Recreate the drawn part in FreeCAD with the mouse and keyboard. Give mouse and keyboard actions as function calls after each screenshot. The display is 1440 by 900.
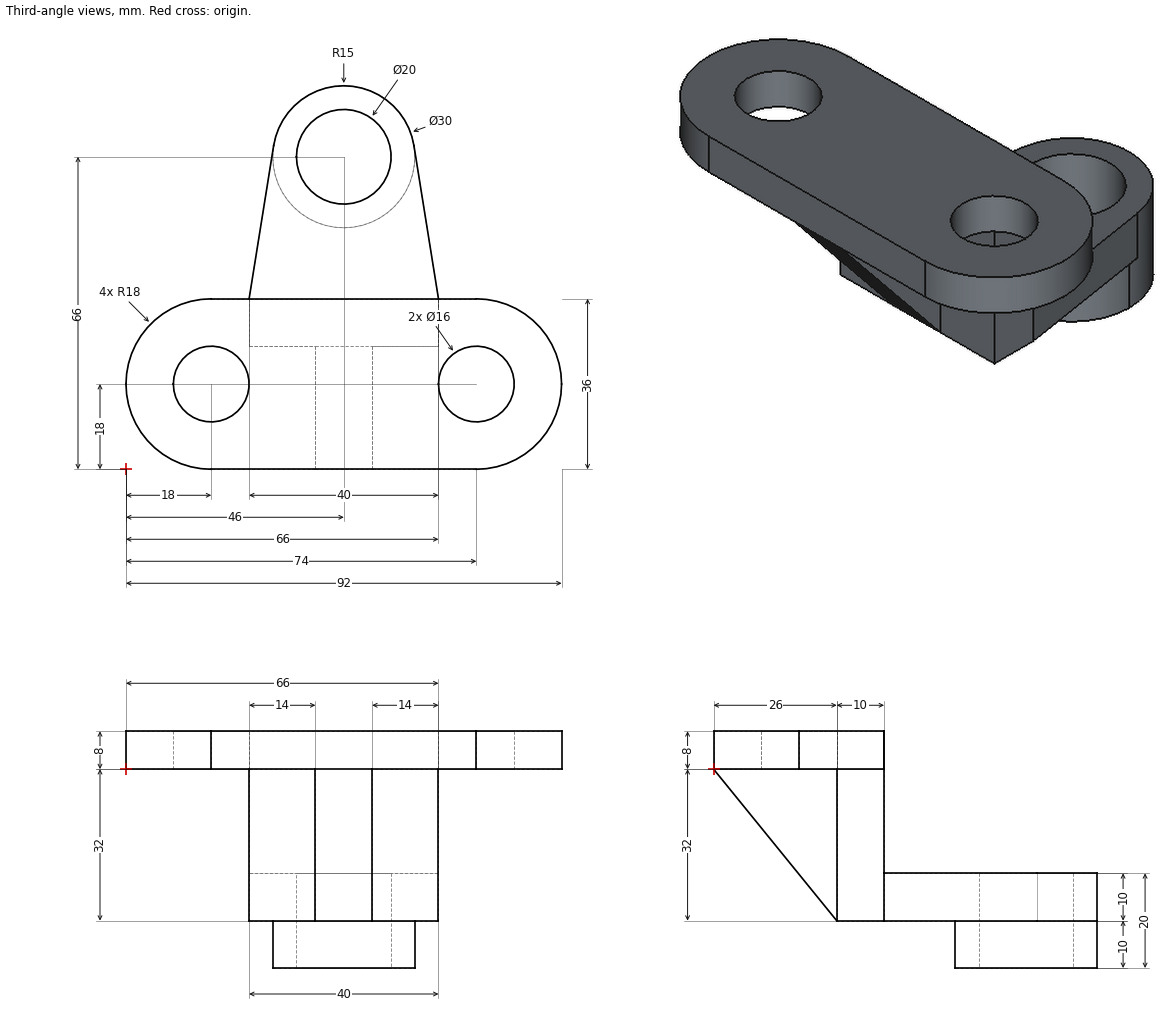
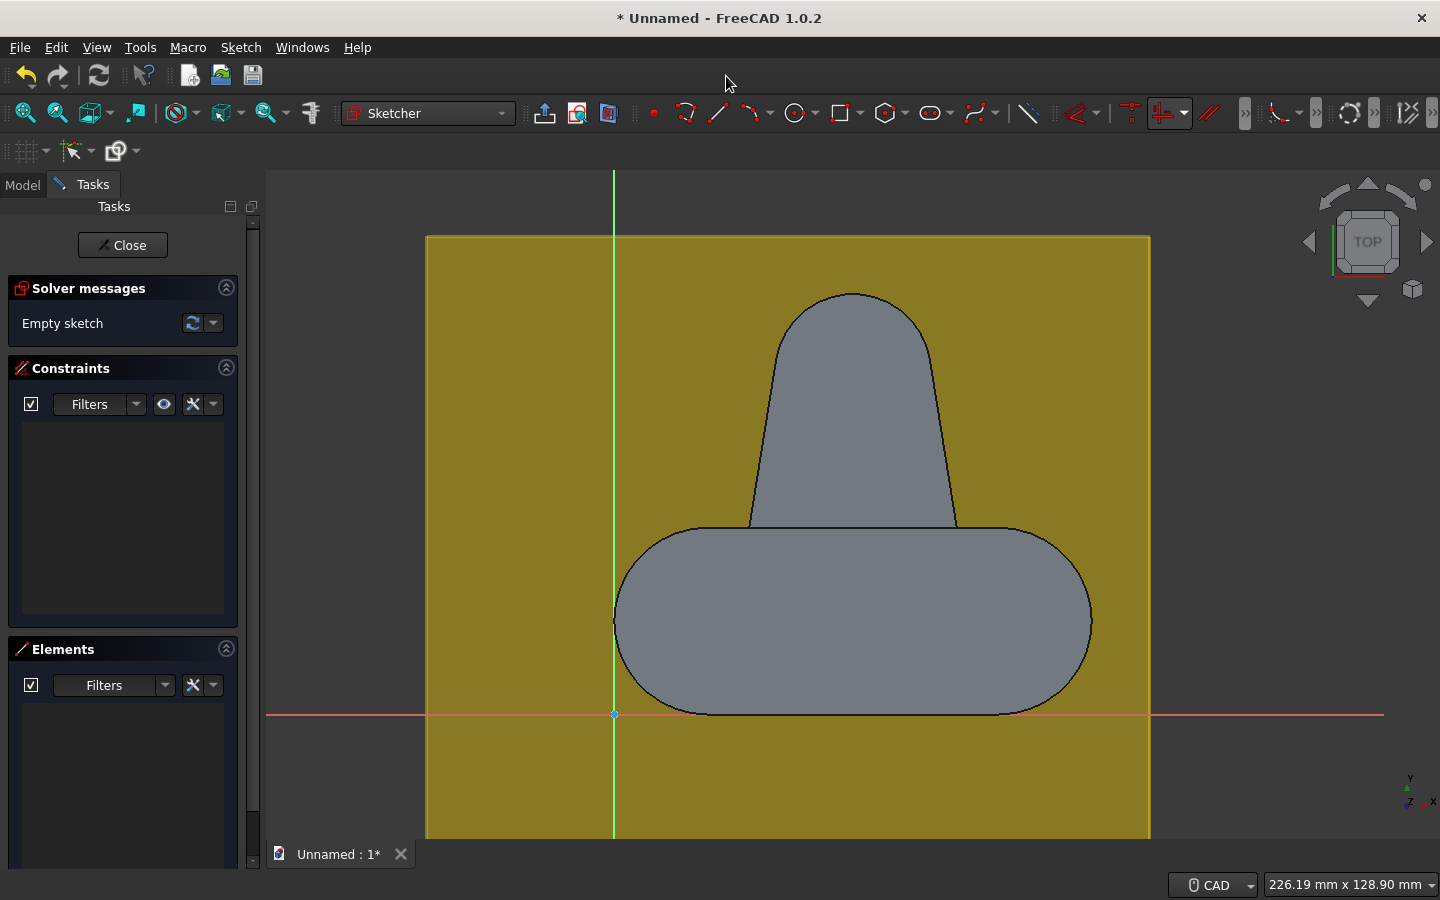
click(610, 114)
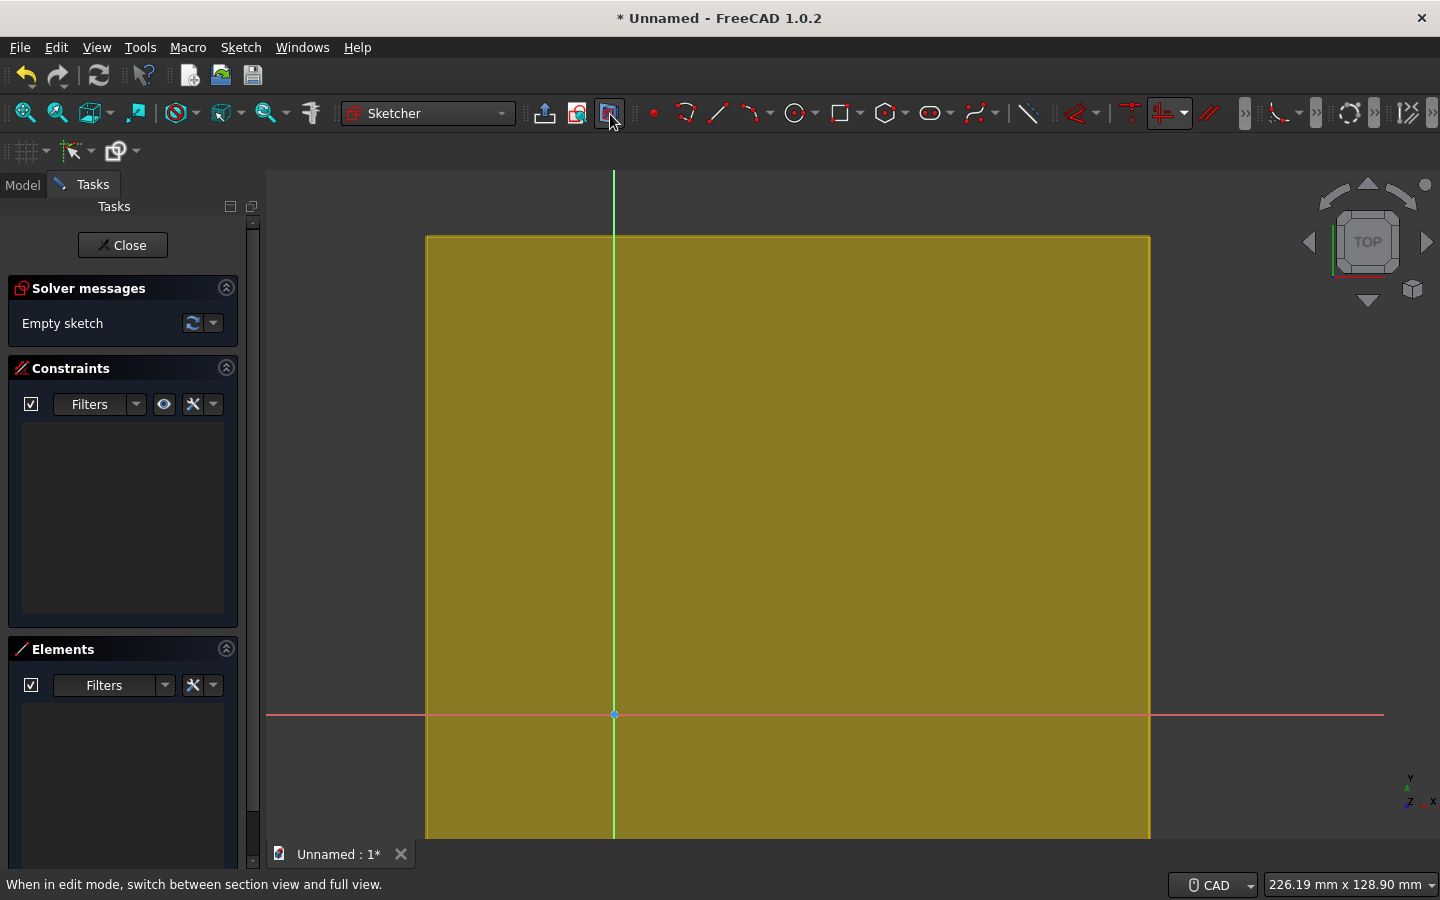
scroll(893, 295, up, 5)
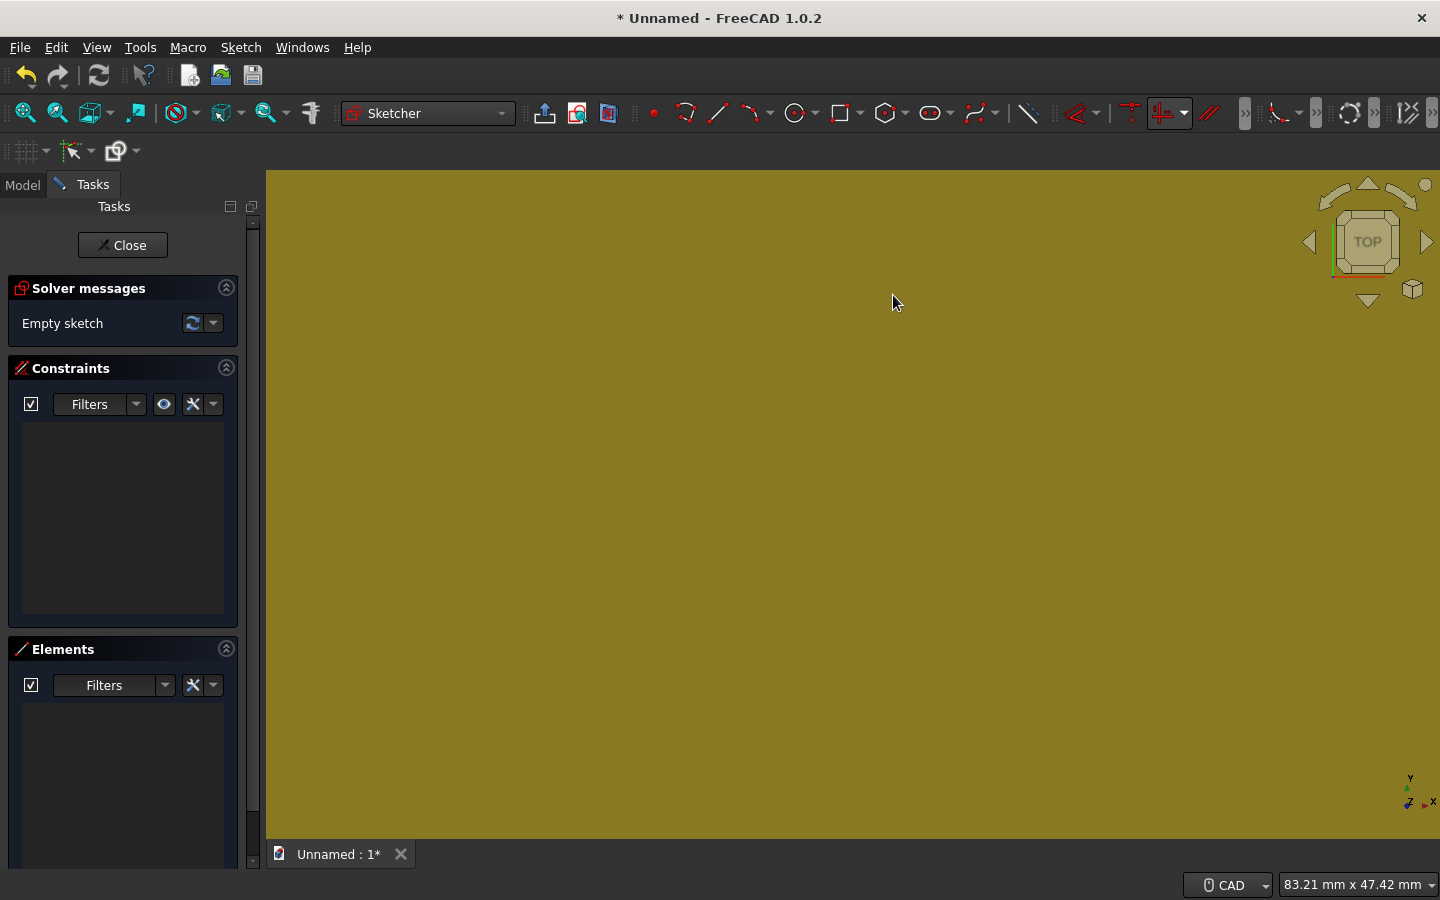
click(796, 114)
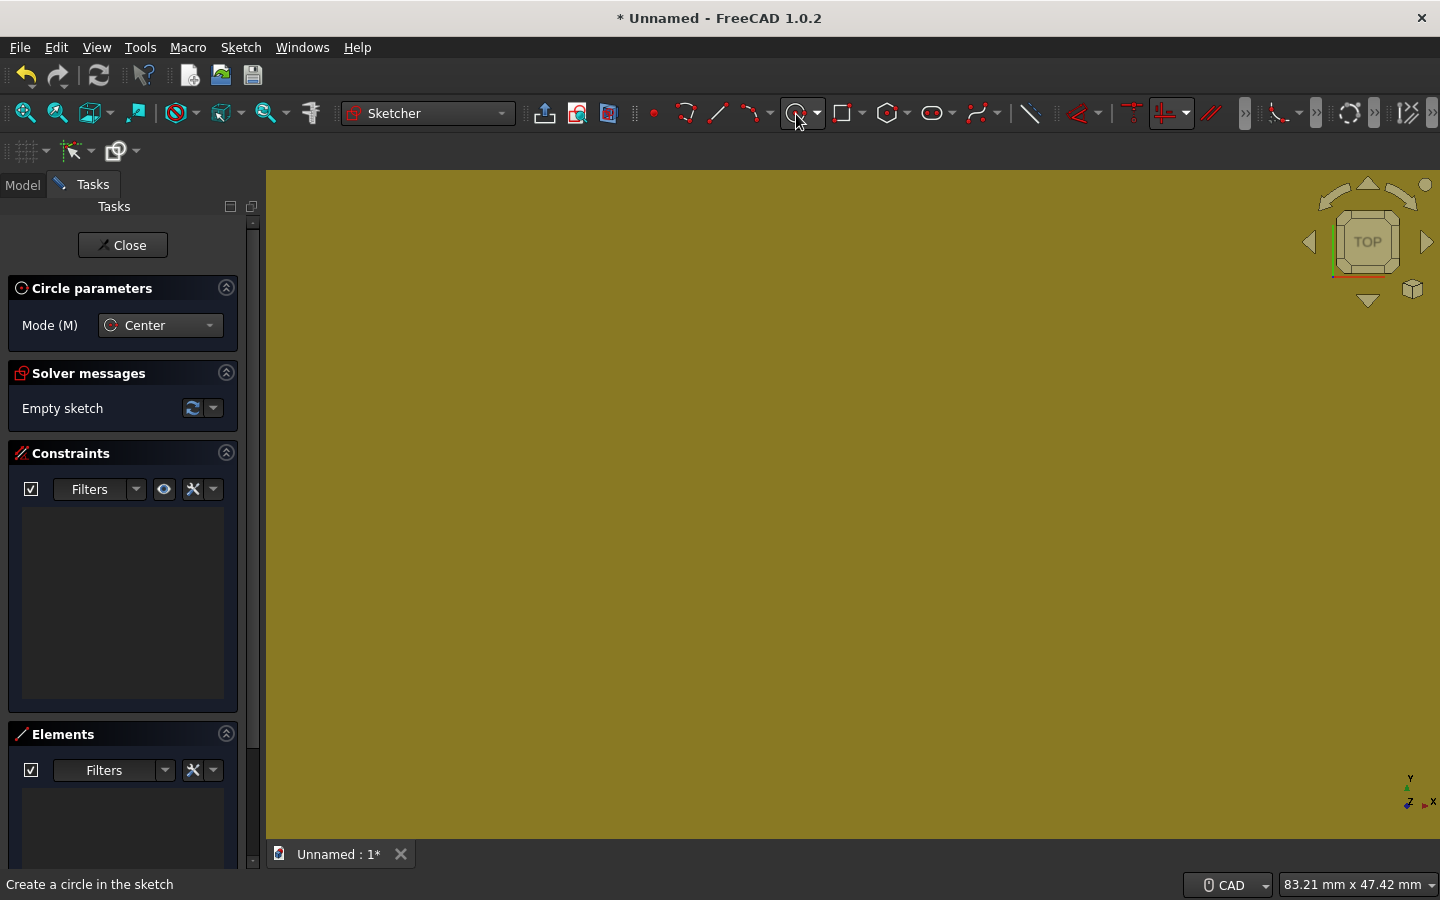
click(783, 504)
move(933, 354)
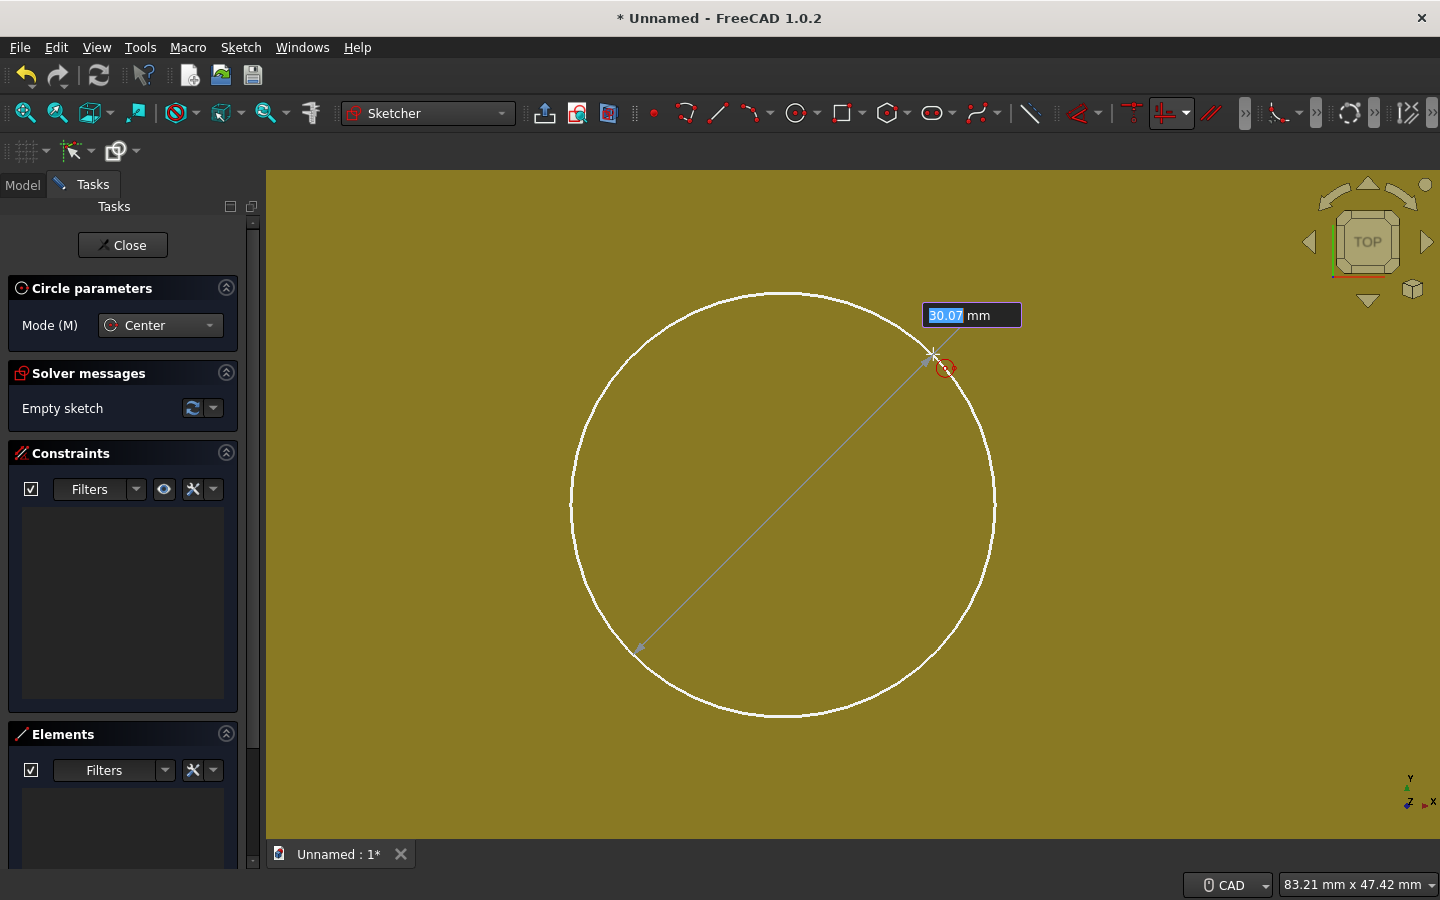
text(30)
key(Return)
key(Escape)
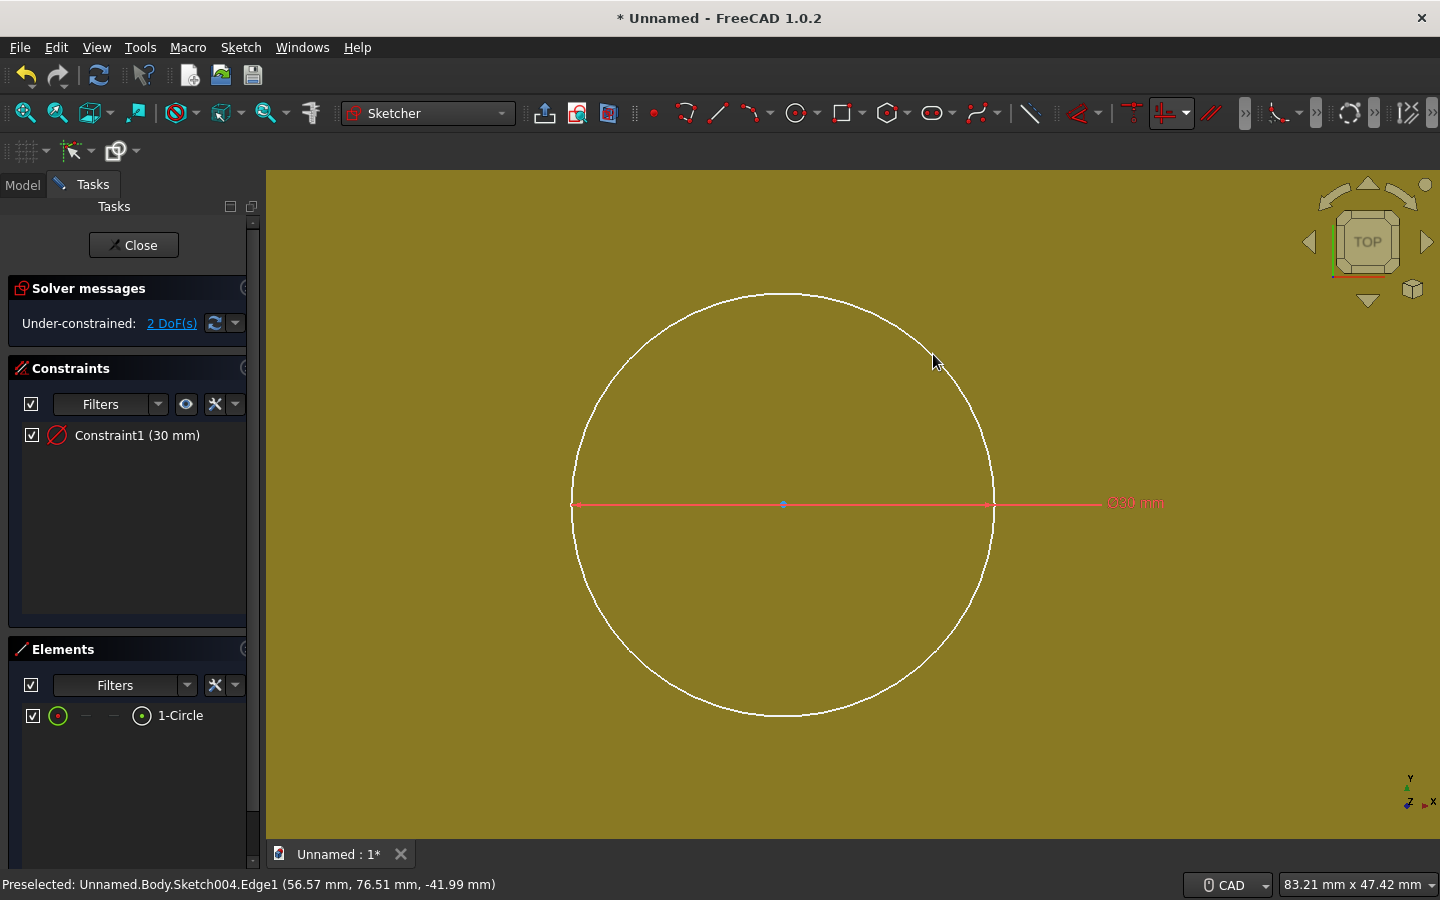
click(1078, 114)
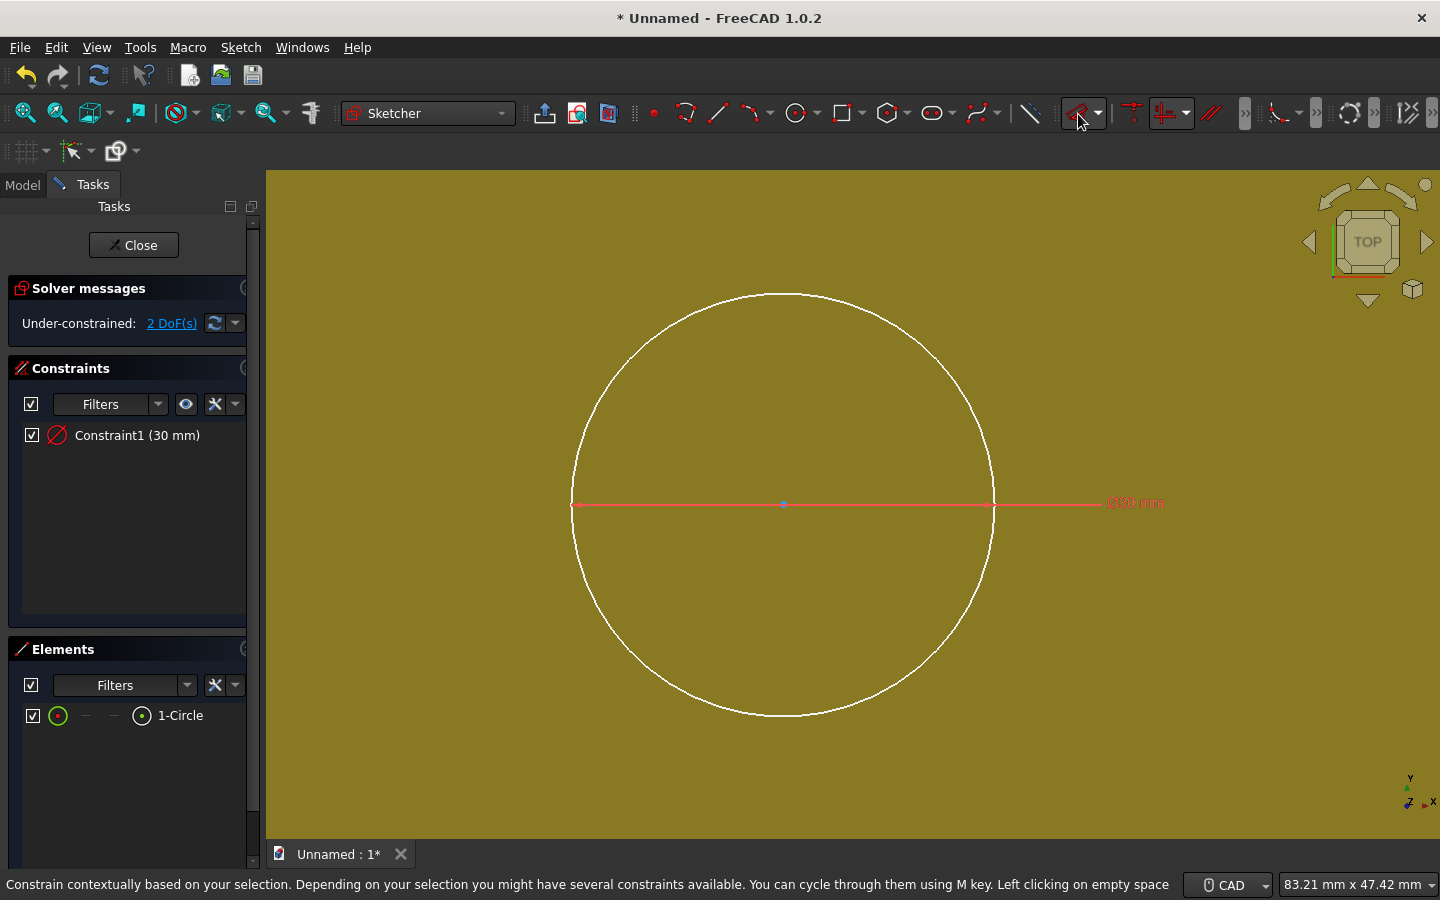
click(783, 505)
click(538, 471)